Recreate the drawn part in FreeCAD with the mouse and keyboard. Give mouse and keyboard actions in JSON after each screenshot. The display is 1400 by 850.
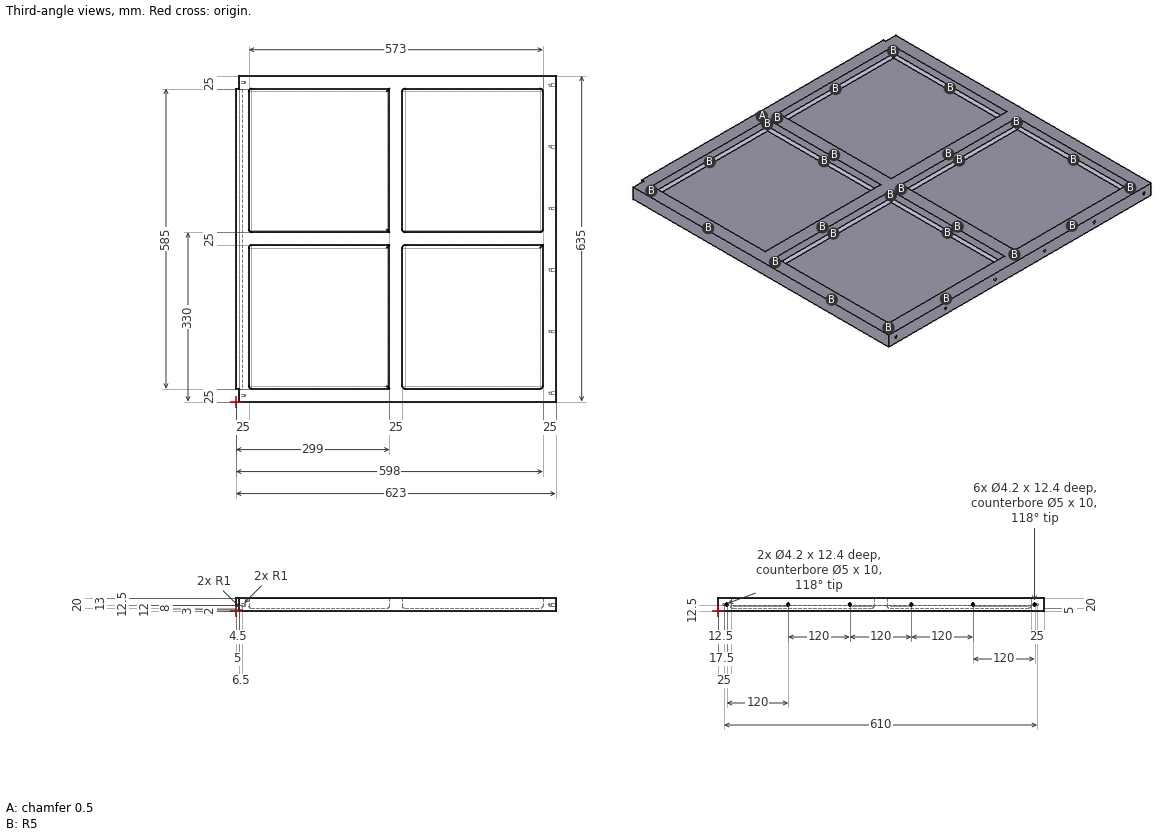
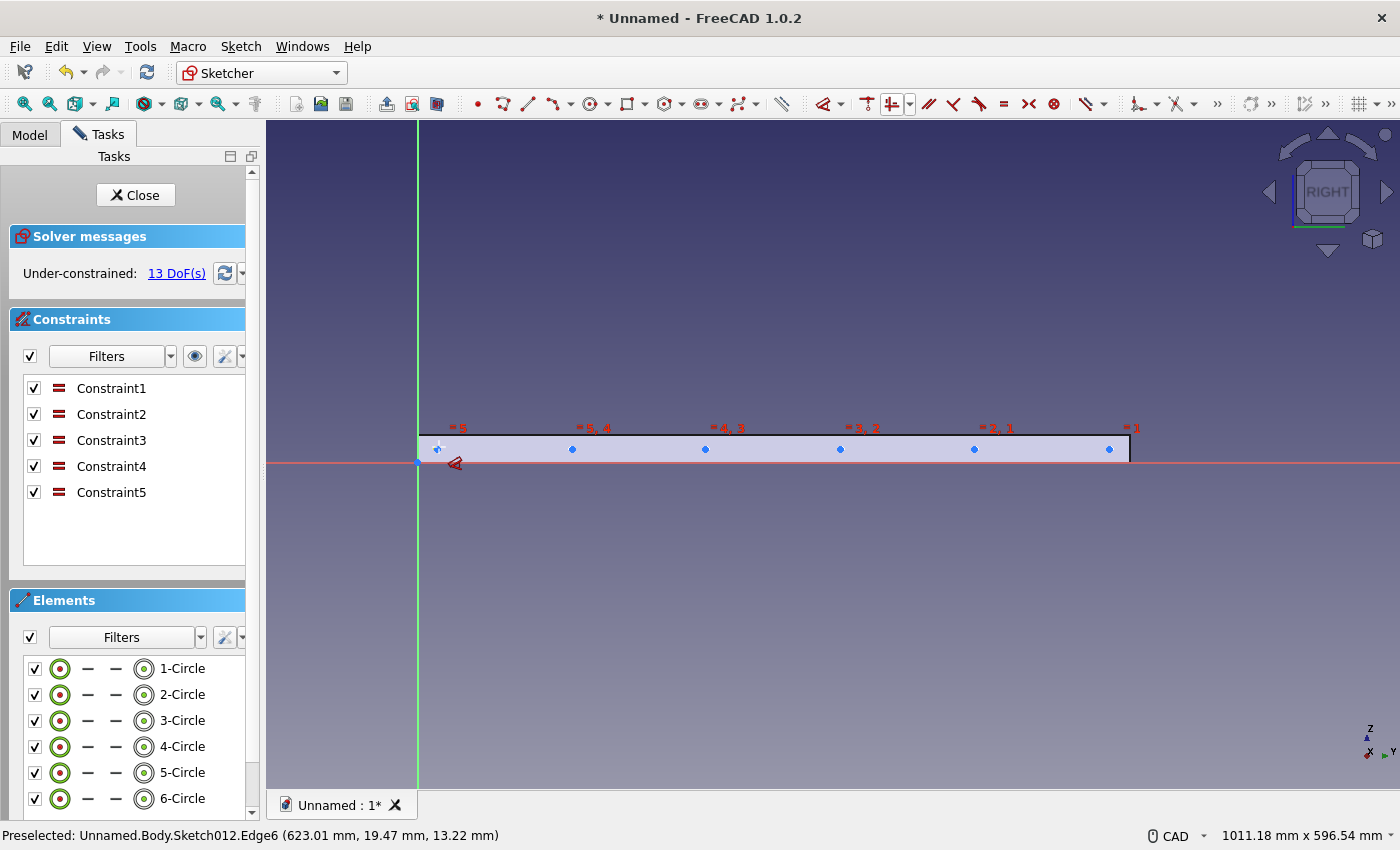
{"action": "scroll", "coordinate": [1112, 447], "scroll_direction": "up", "scroll_amount": 11}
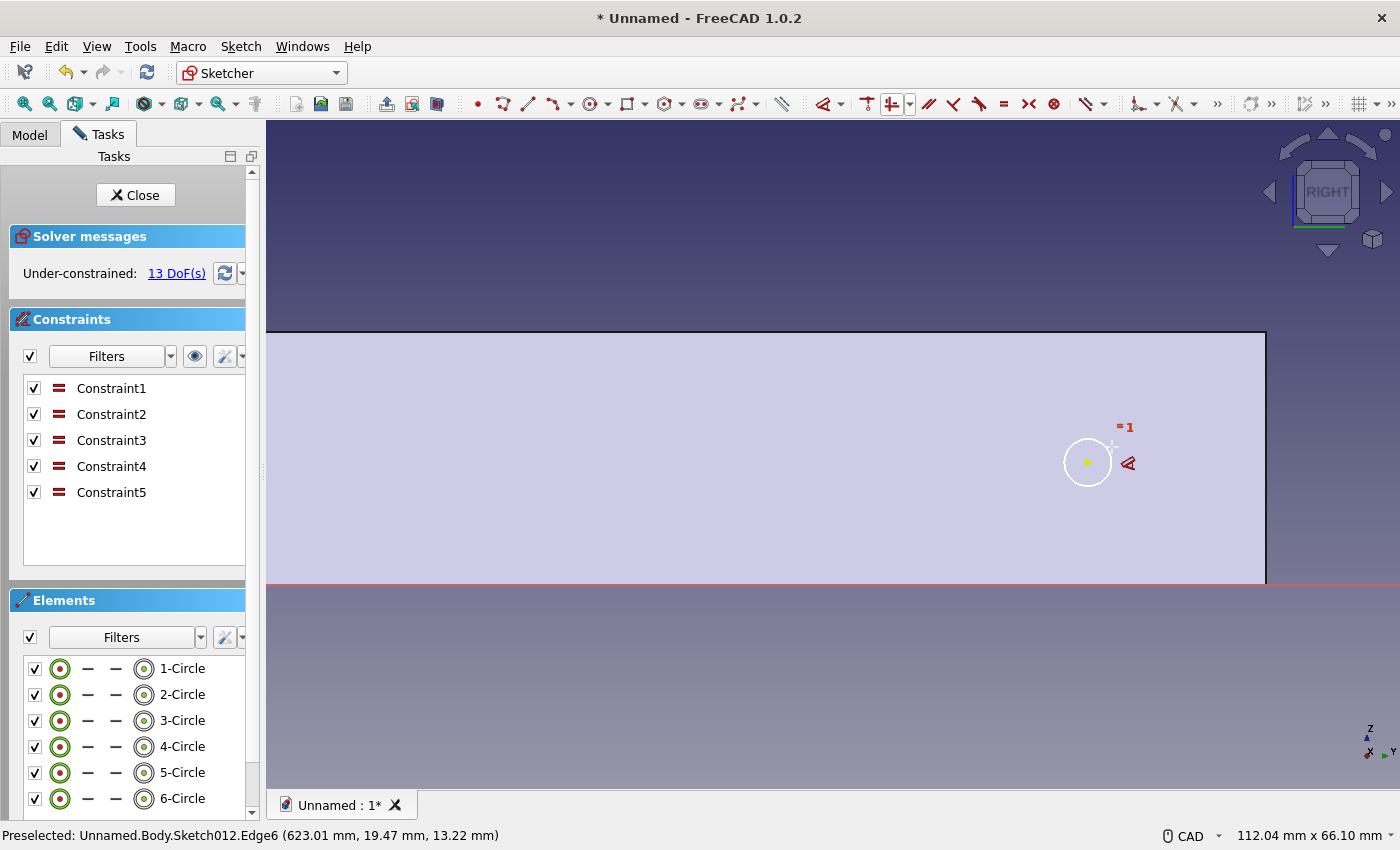
{"action": "left_click", "coordinate": [1105, 446]}
{"action": "left_click", "coordinate": [1128, 424]}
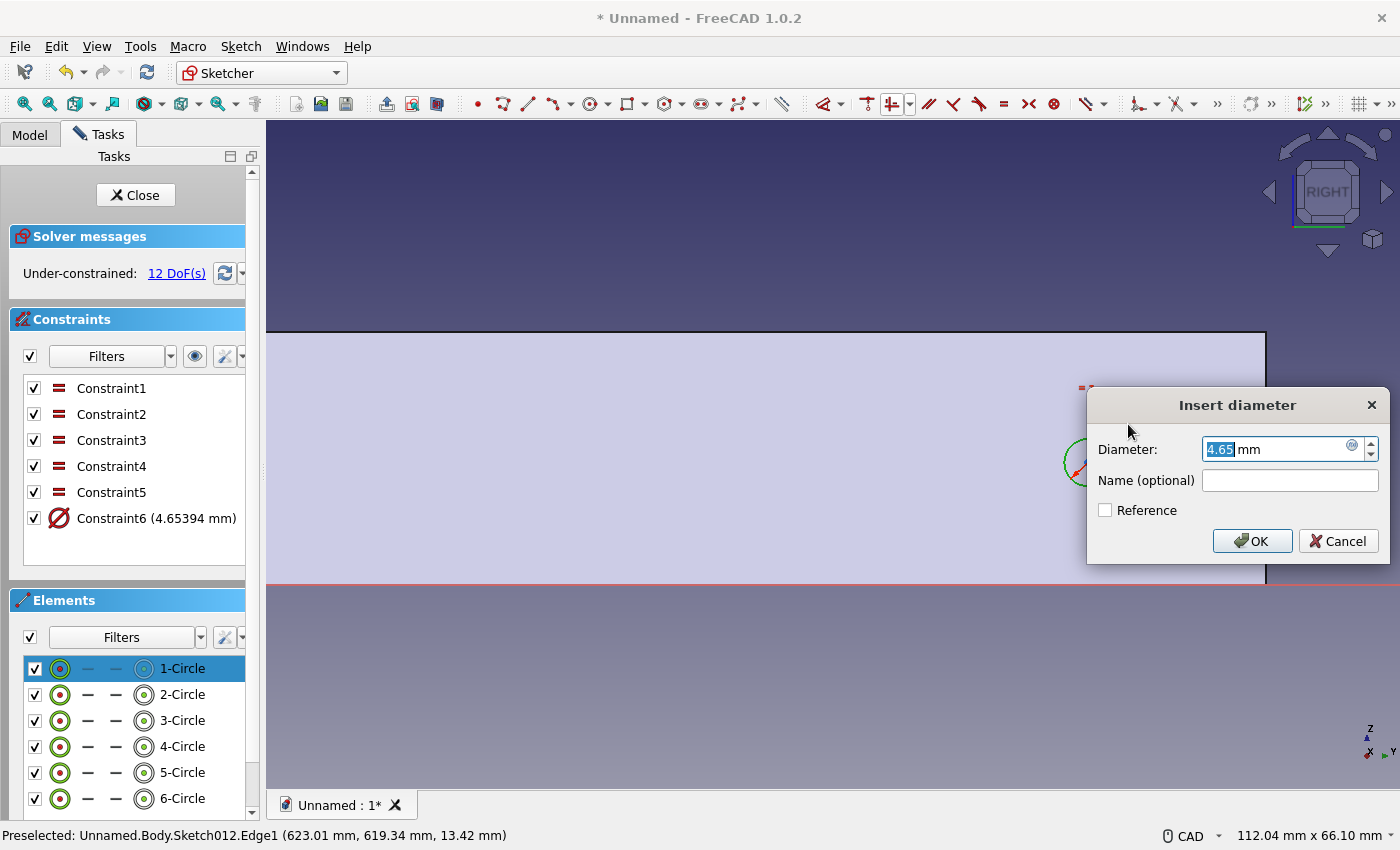
{"action": "type", "text": "4.2"}
{"action": "key", "text": "Return"}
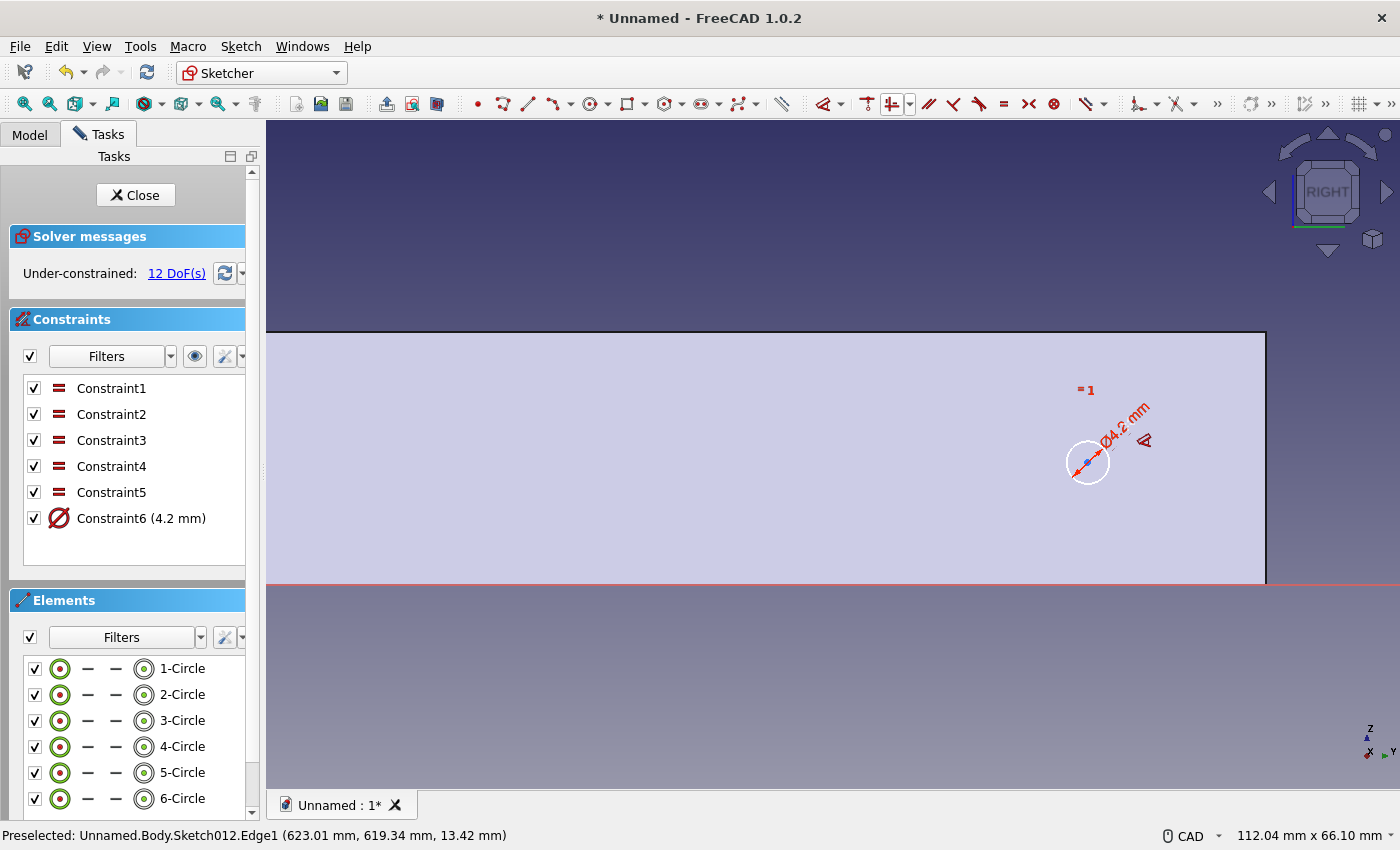
{"action": "scroll", "coordinate": [1112, 447], "scroll_direction": "down", "scroll_amount": 11}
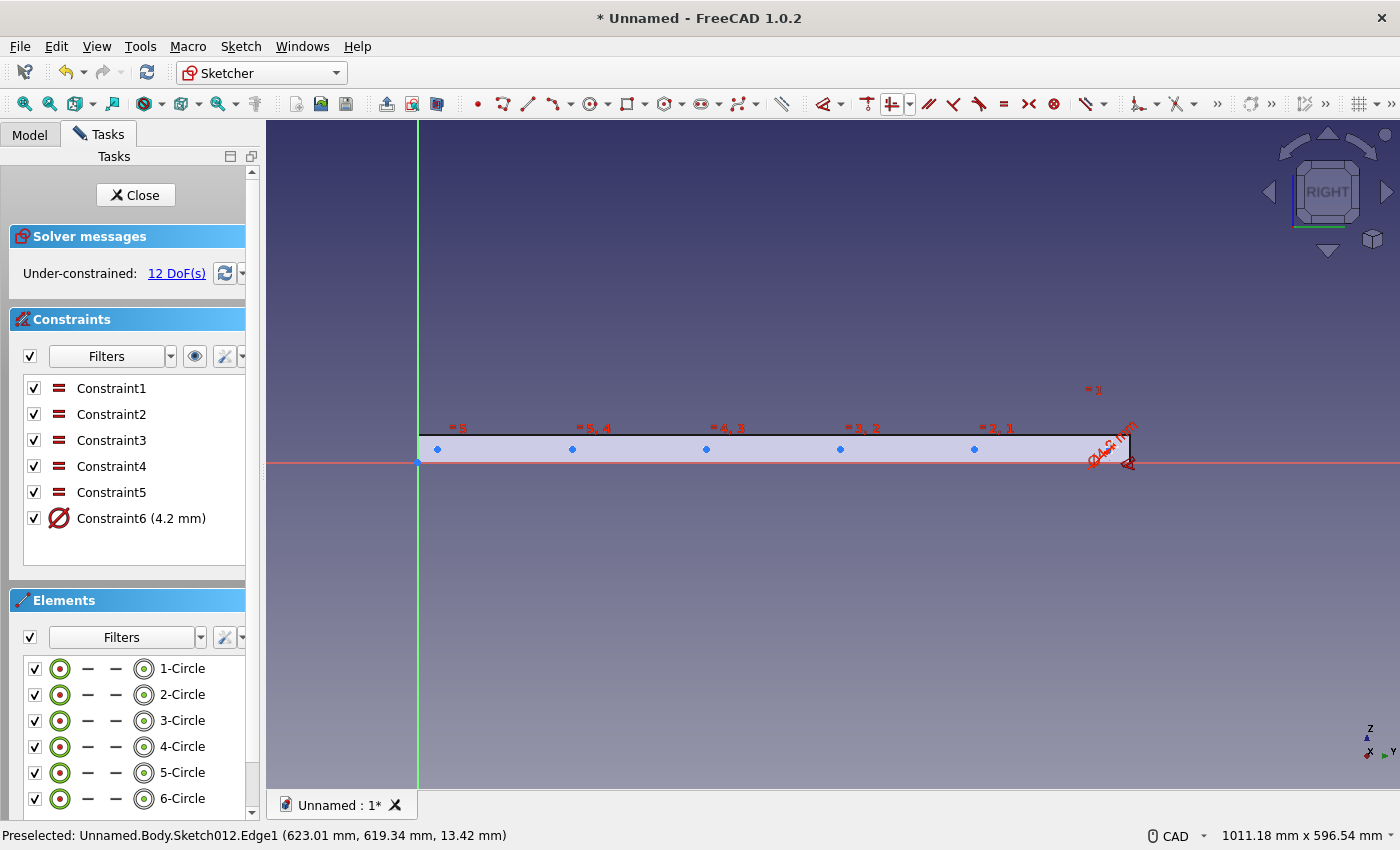
{"action": "scroll", "coordinate": [1110, 449], "scroll_direction": "up", "scroll_amount": 6}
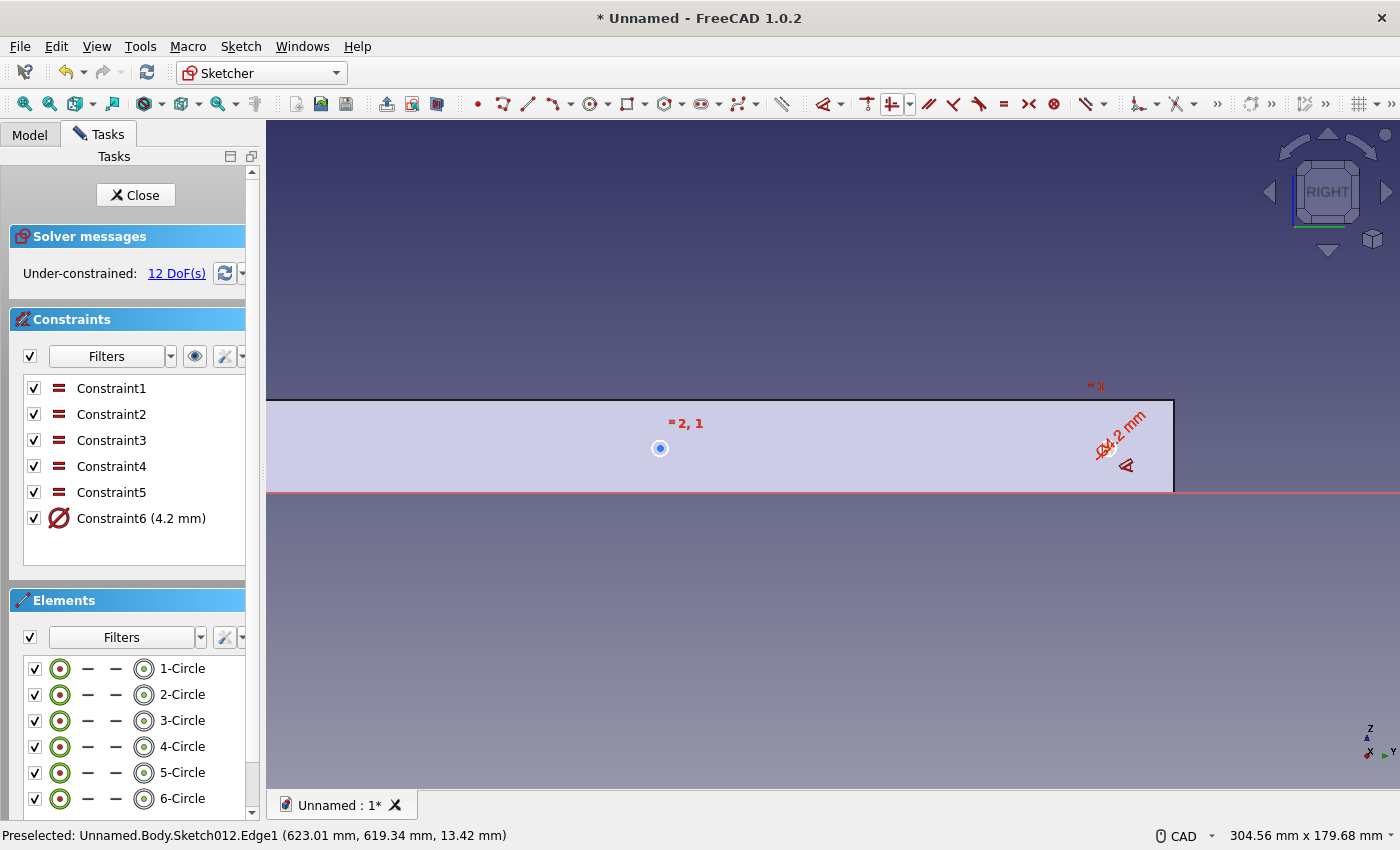
{"action": "left_click", "coordinate": [1108, 448]}
{"action": "left_click", "coordinate": [1142, 471]}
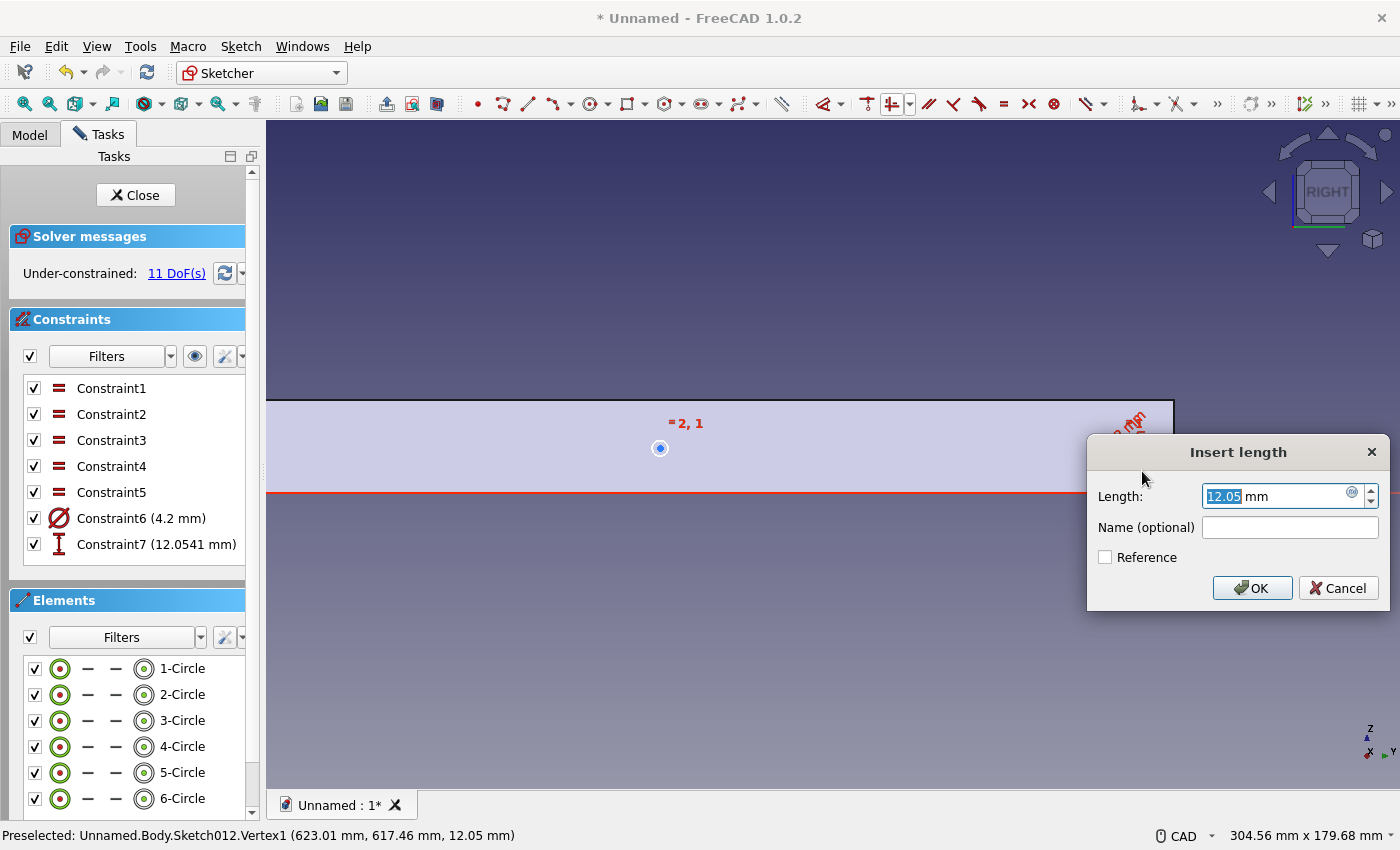
{"action": "type", "text": "12.5"}
{"action": "key", "text": "Return"}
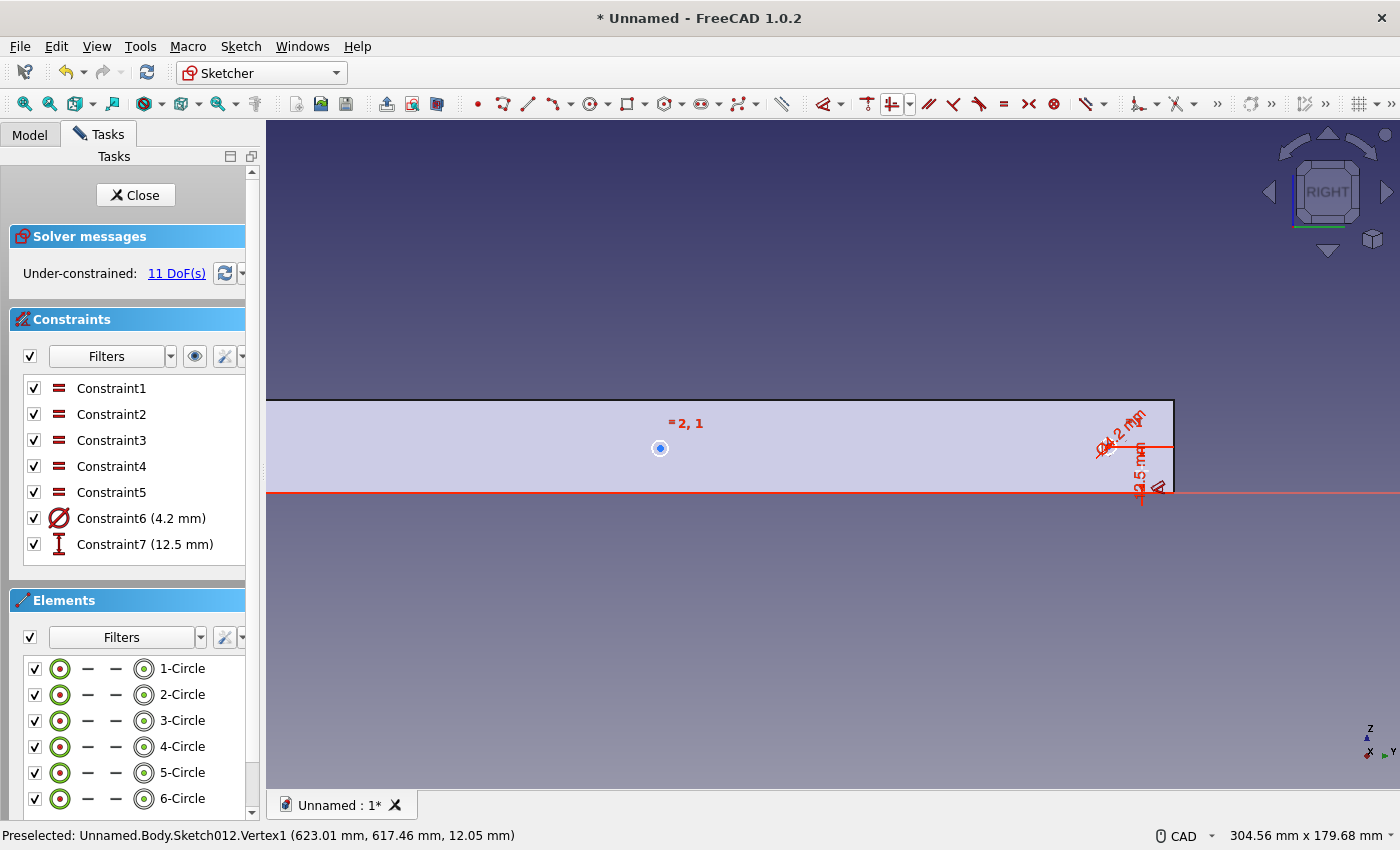
{"action": "left_click", "coordinate": [660, 448]}
{"action": "left_click", "coordinate": [694, 471]}